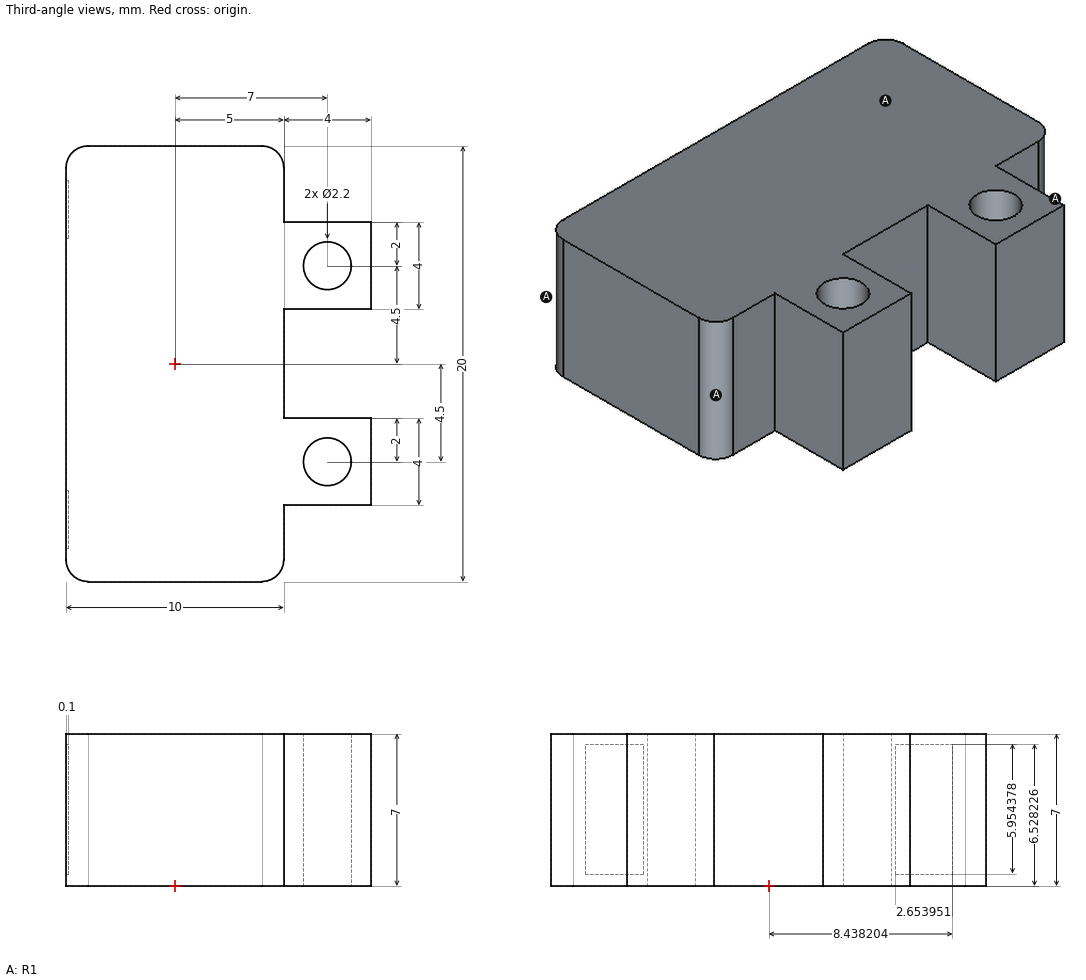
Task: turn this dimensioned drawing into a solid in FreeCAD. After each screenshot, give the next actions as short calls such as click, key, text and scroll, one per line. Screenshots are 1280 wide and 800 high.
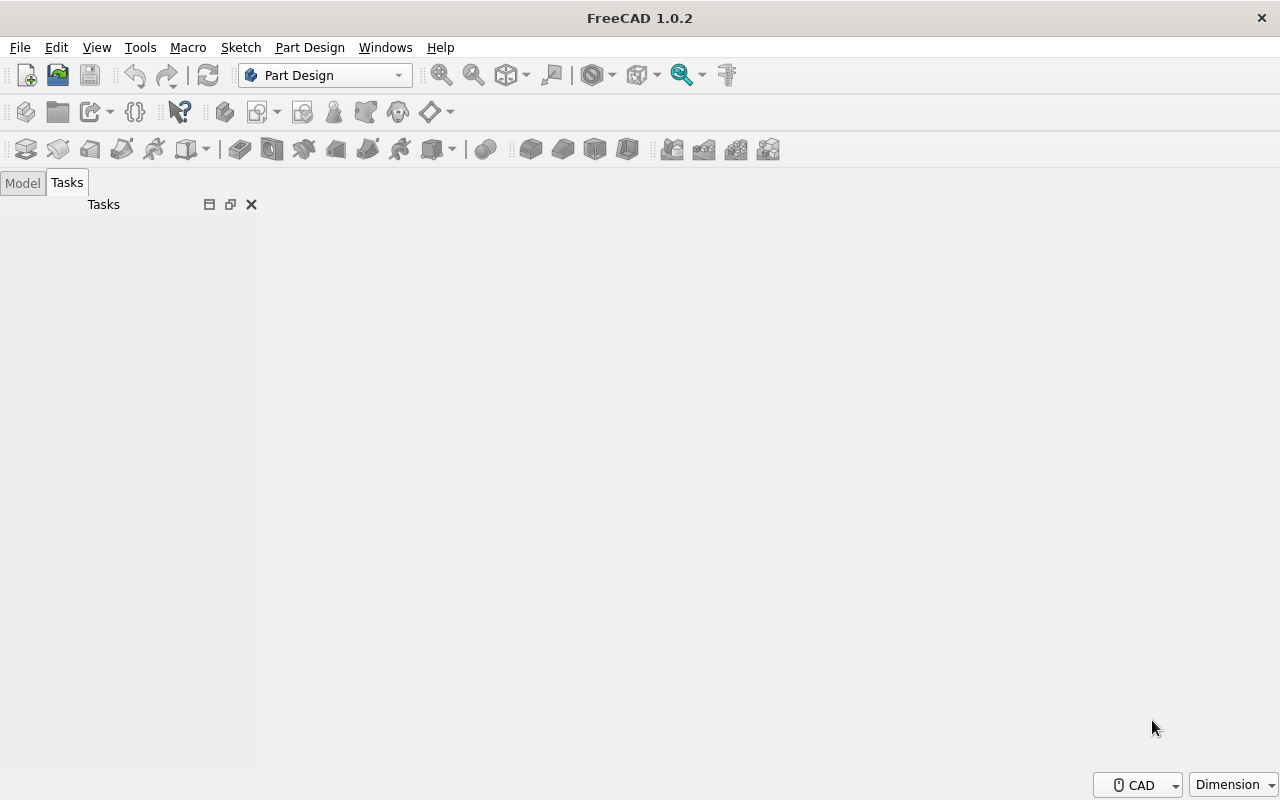
click(26, 76)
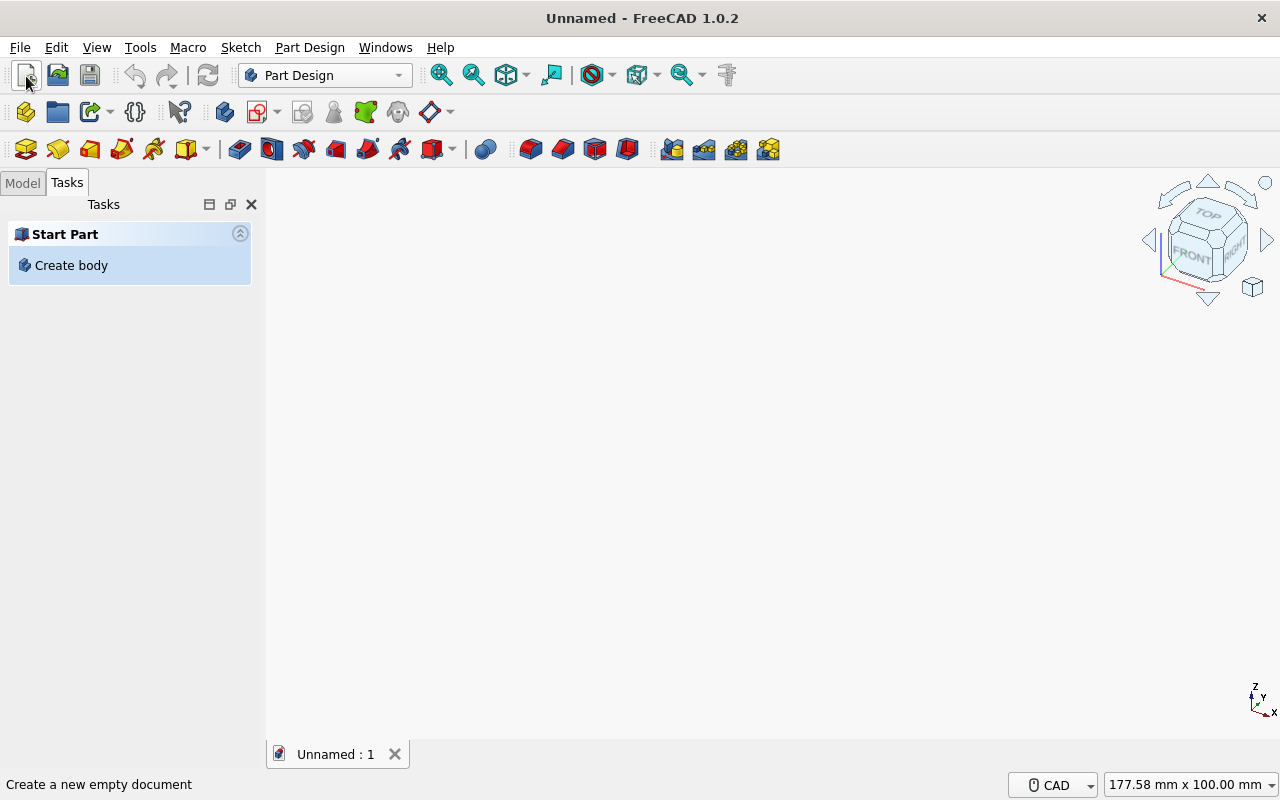
click(258, 112)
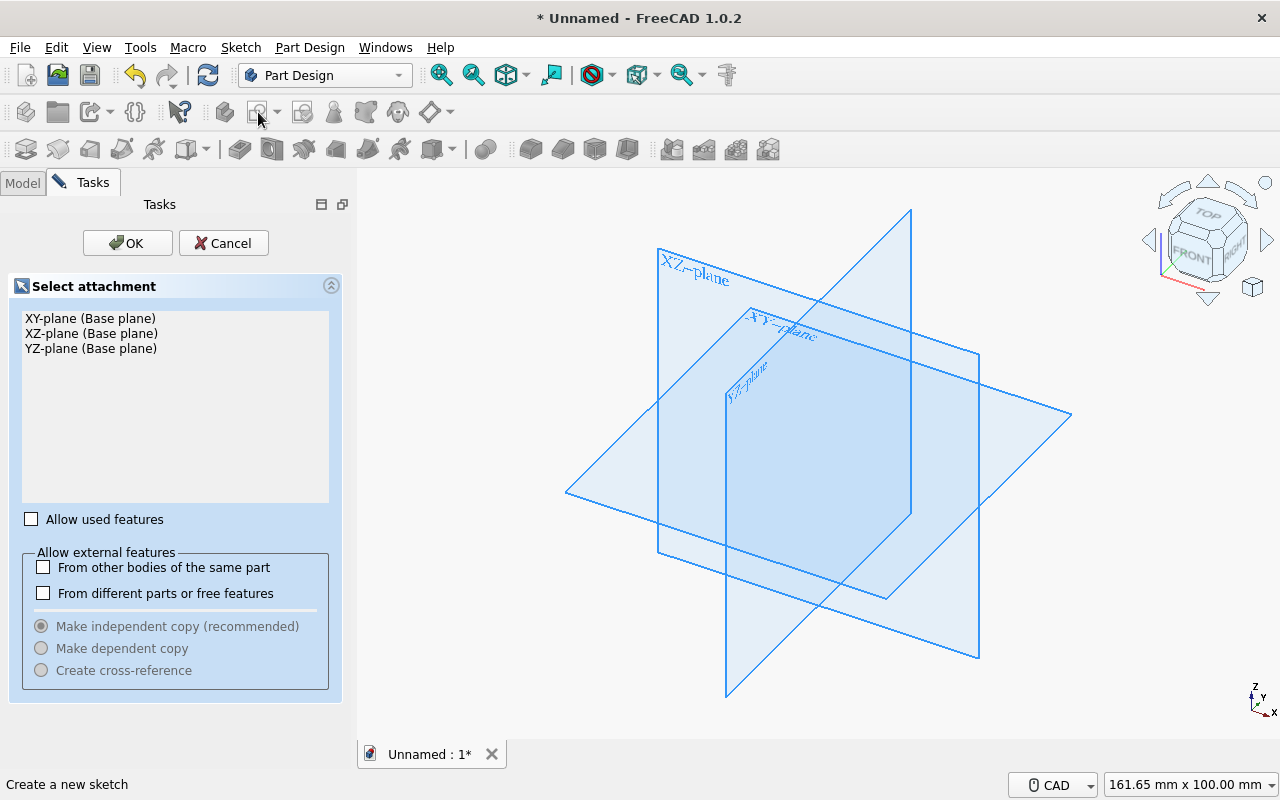
click(82, 318)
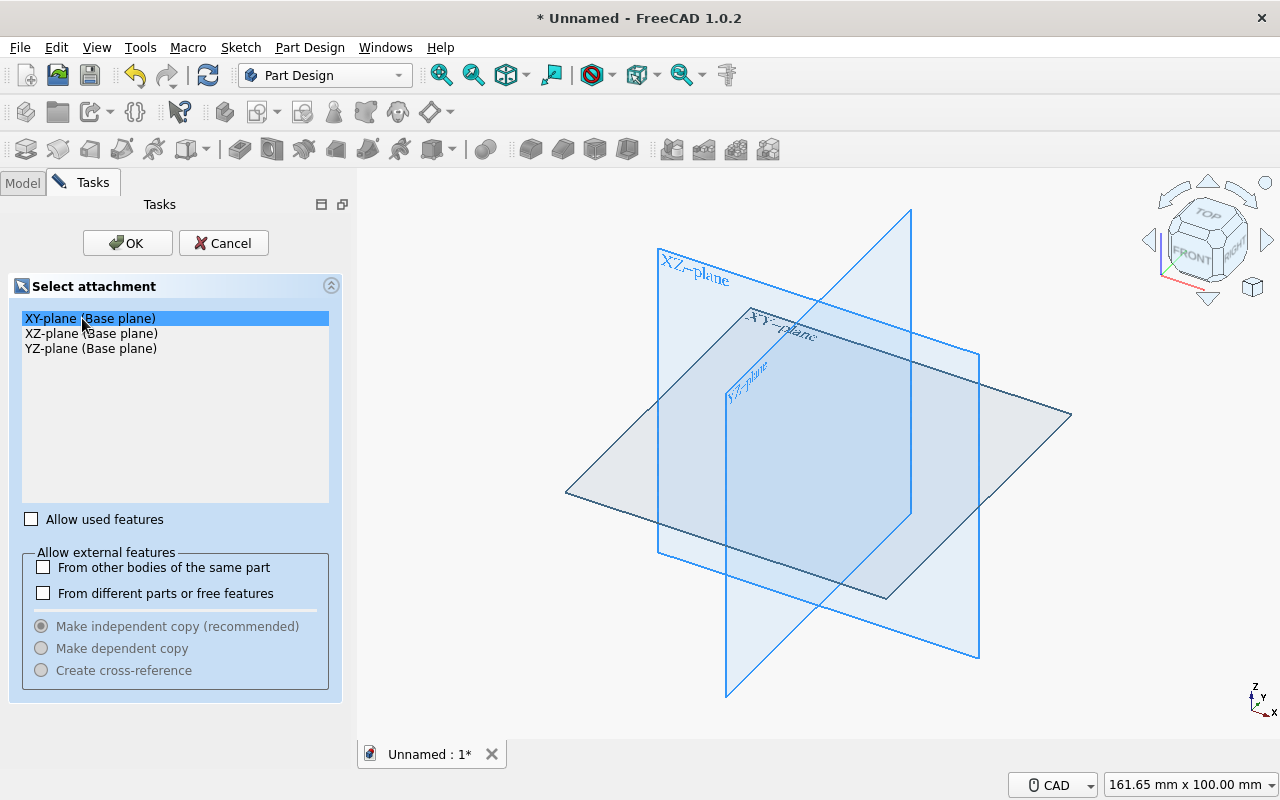
click(128, 243)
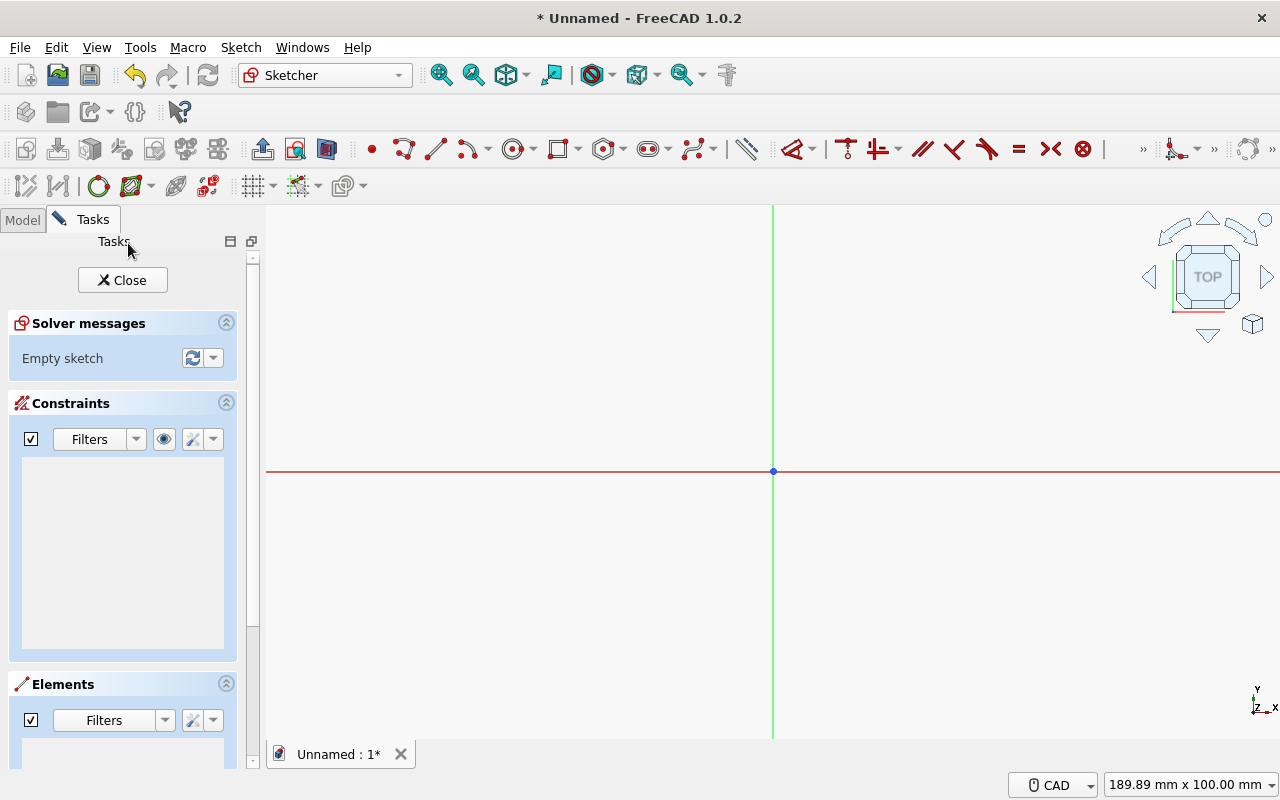
scroll(803, 472, up, 6)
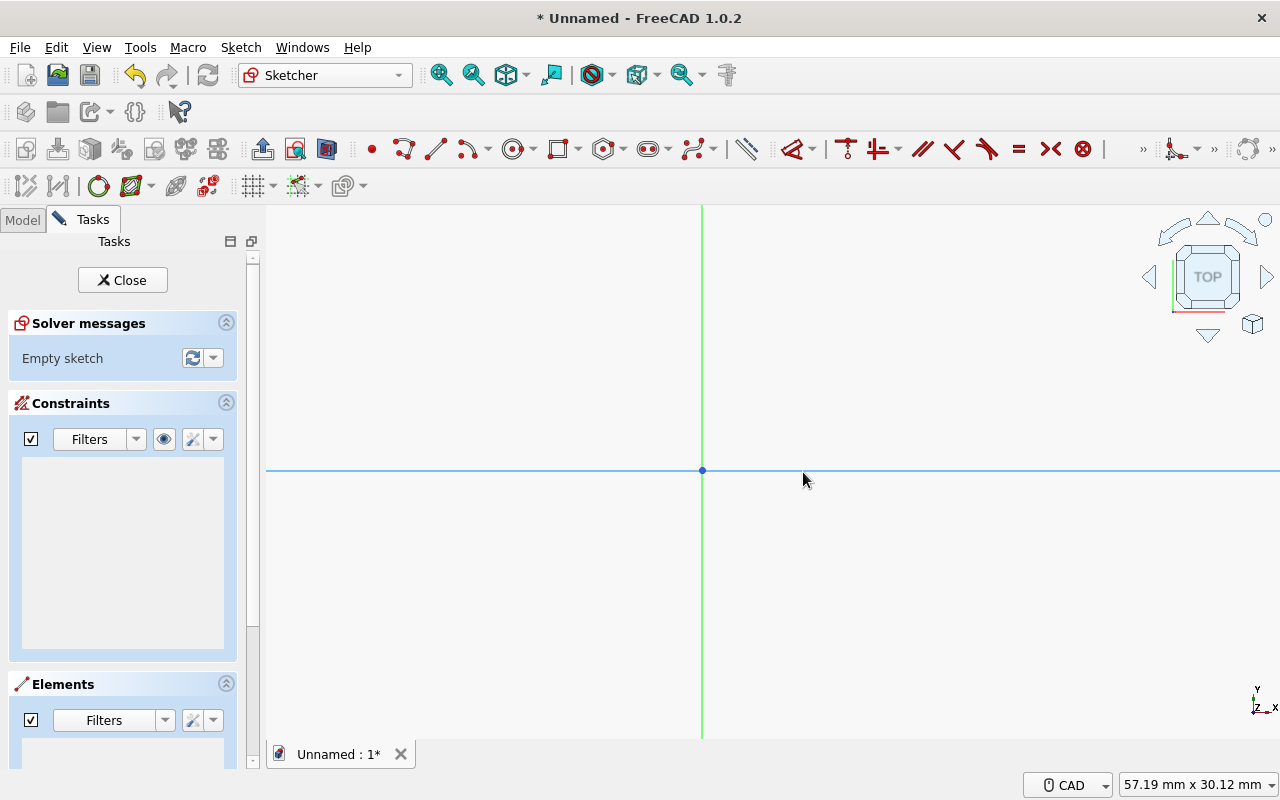
click(580, 150)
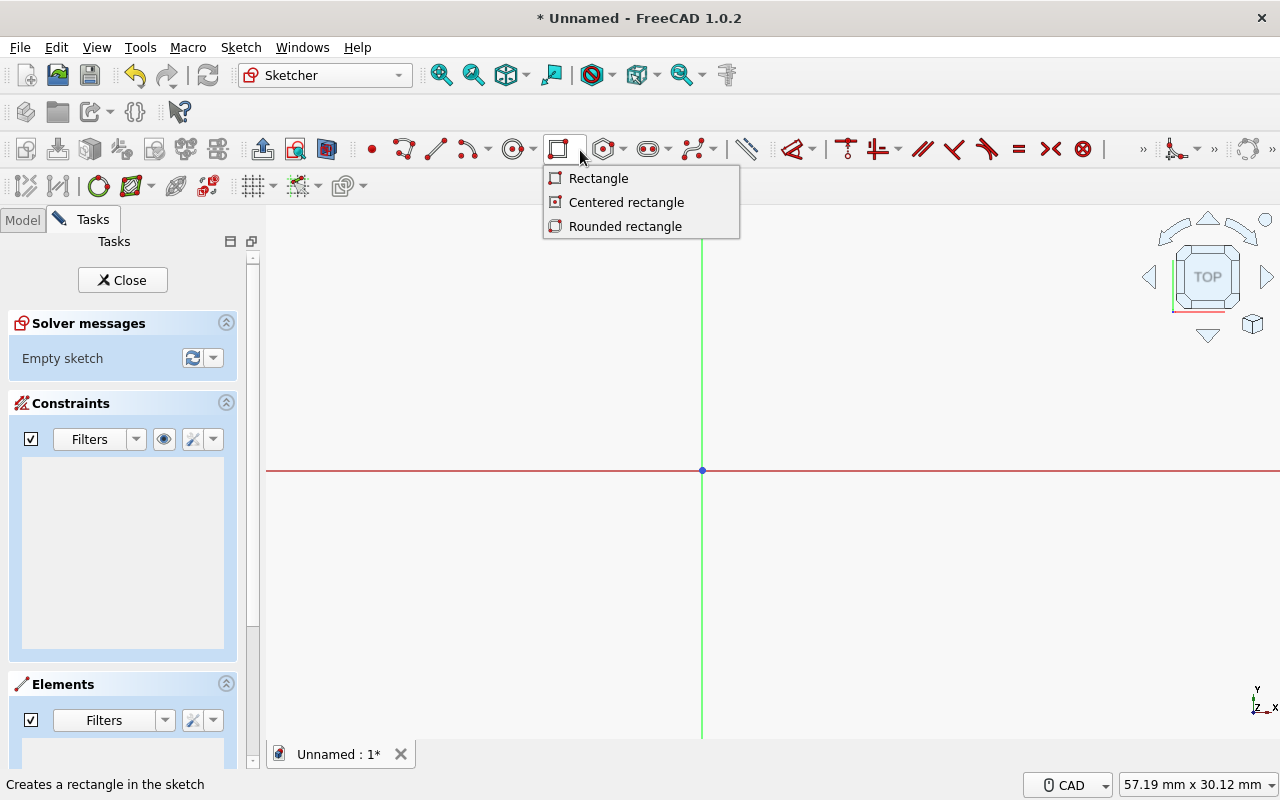
click(642, 202)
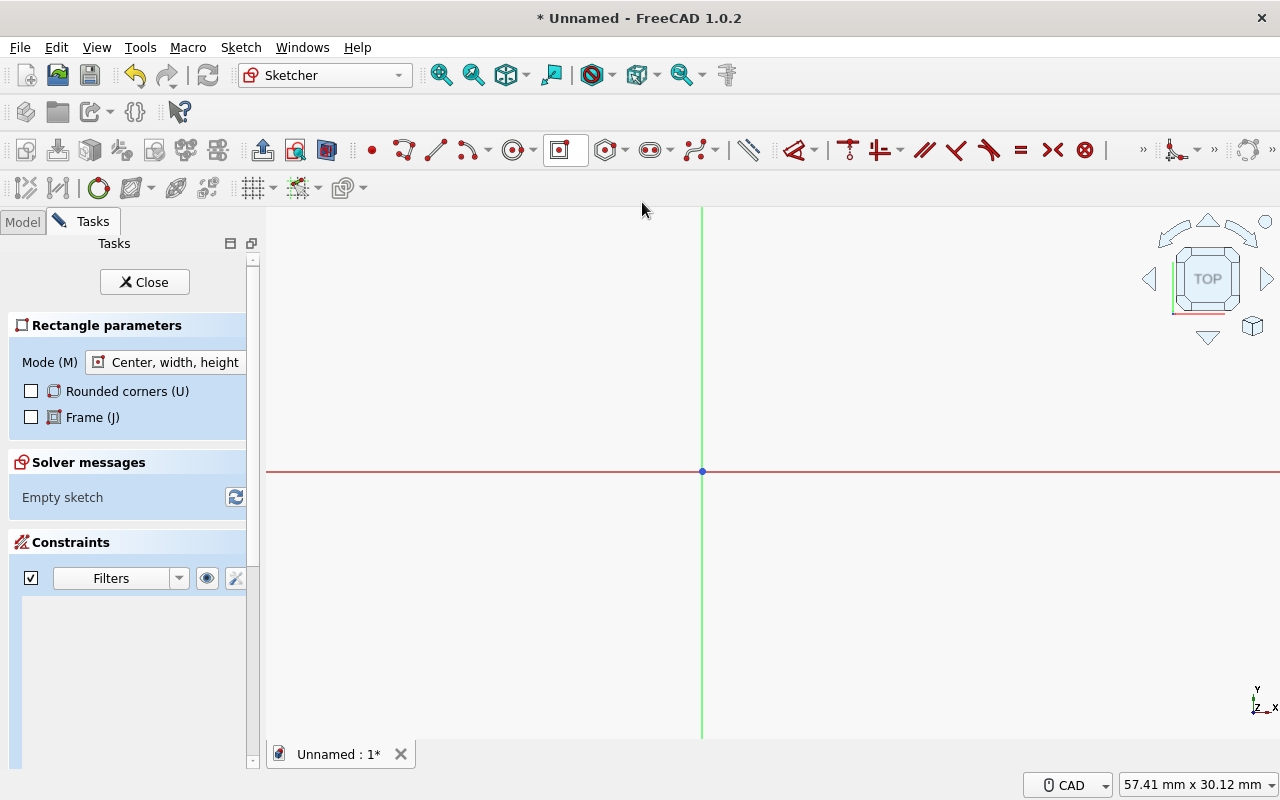
click(702, 472)
click(791, 295)
key(Escape)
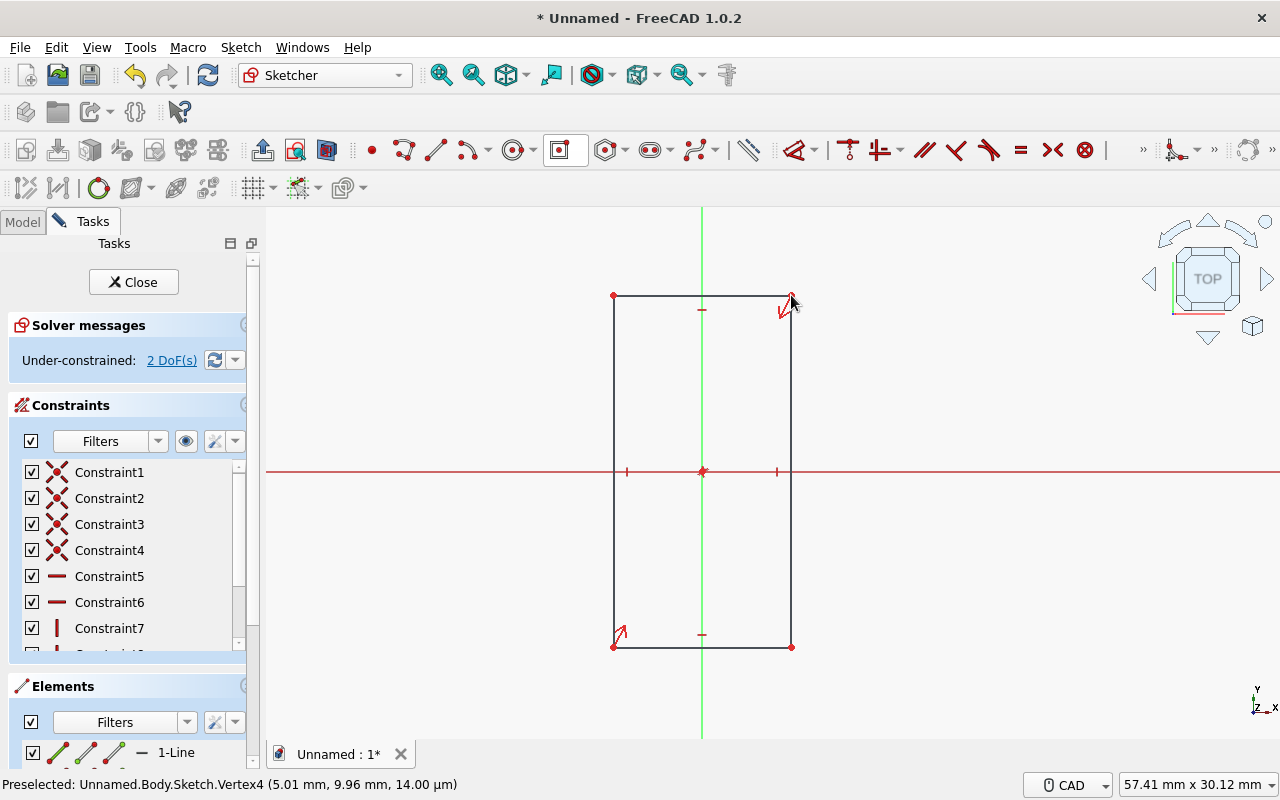
click(667, 648)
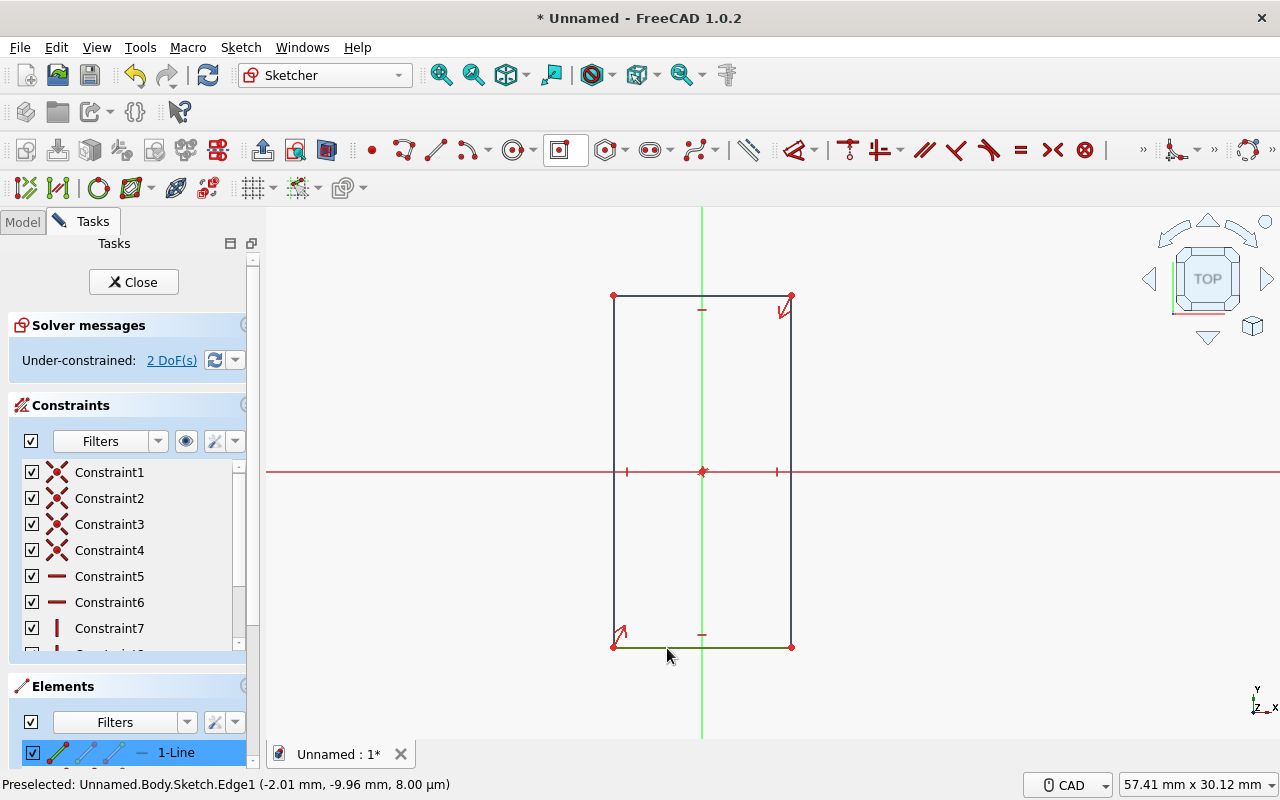
key(l)